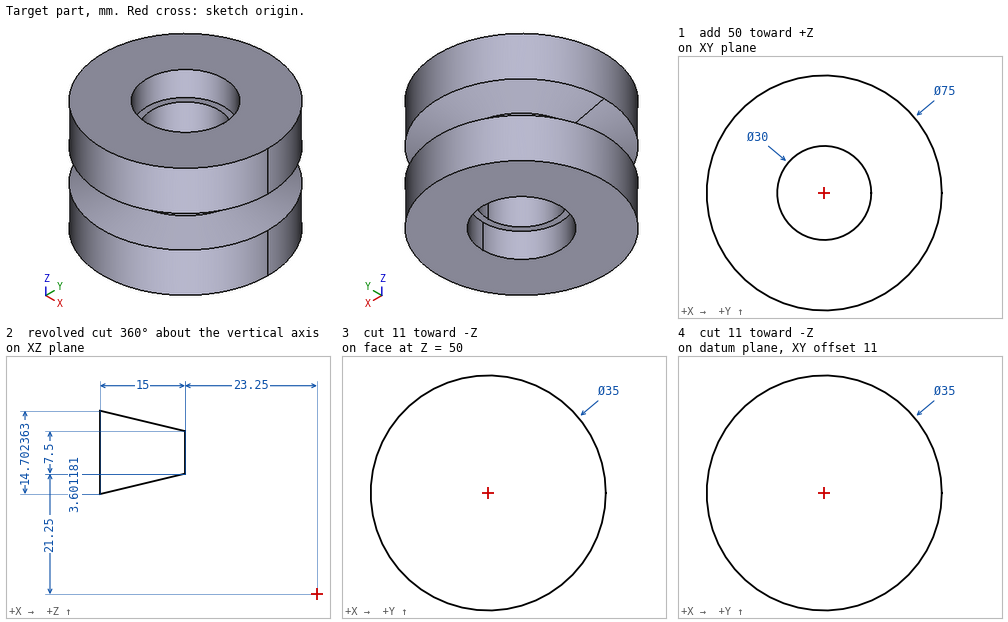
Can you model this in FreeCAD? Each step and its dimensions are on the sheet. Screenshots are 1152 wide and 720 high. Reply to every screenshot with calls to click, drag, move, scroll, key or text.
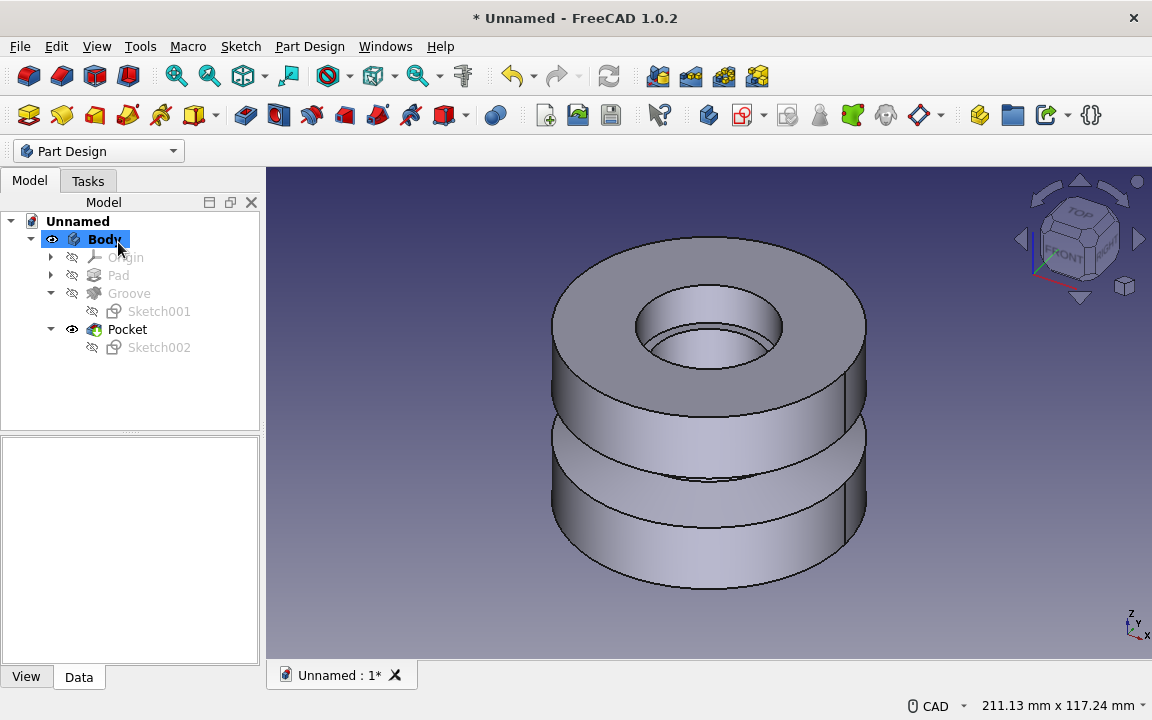
click(51, 257)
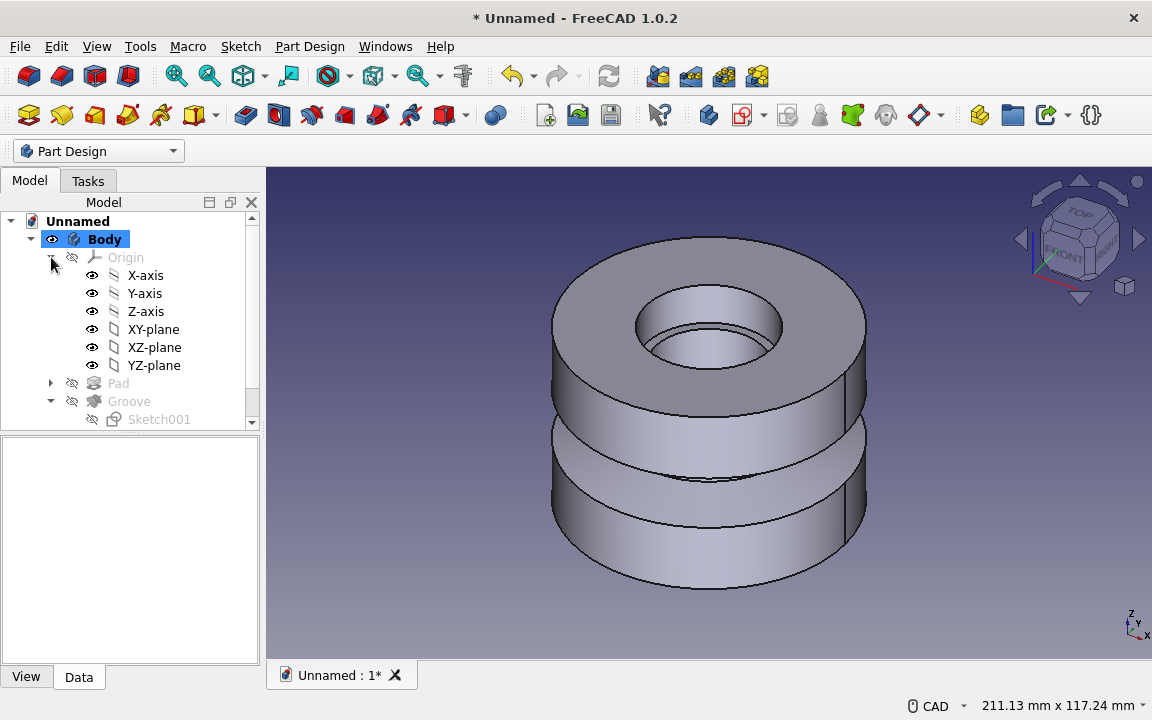
click(137, 329)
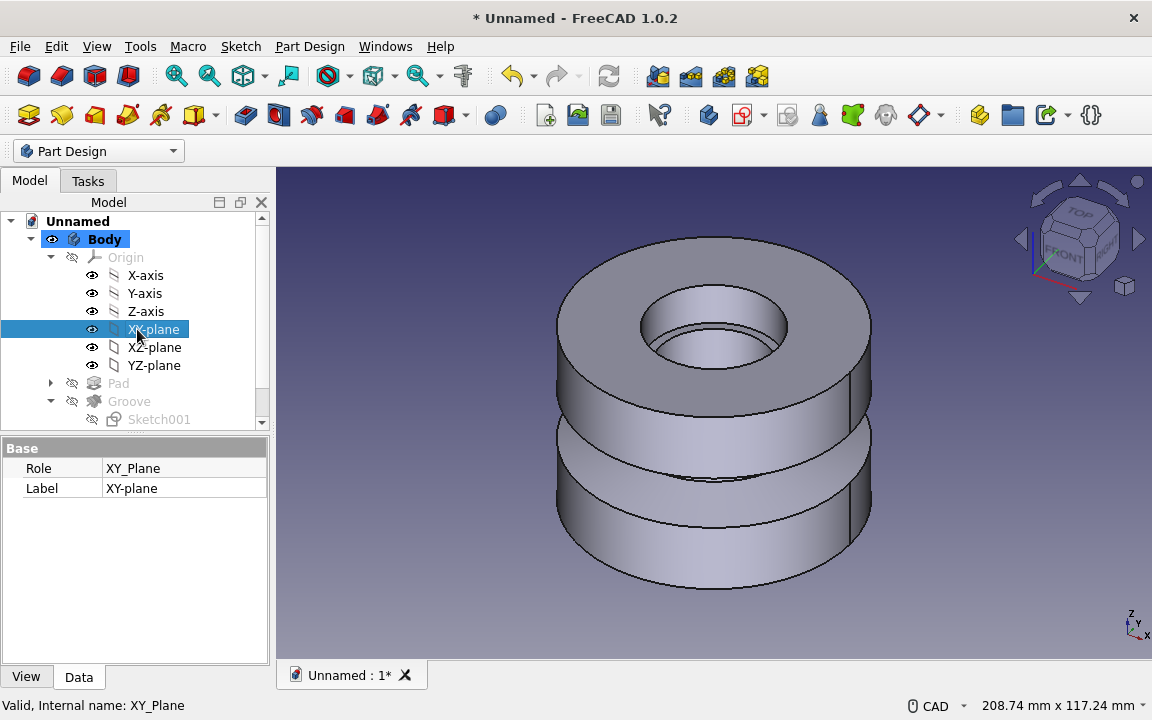
click(918, 116)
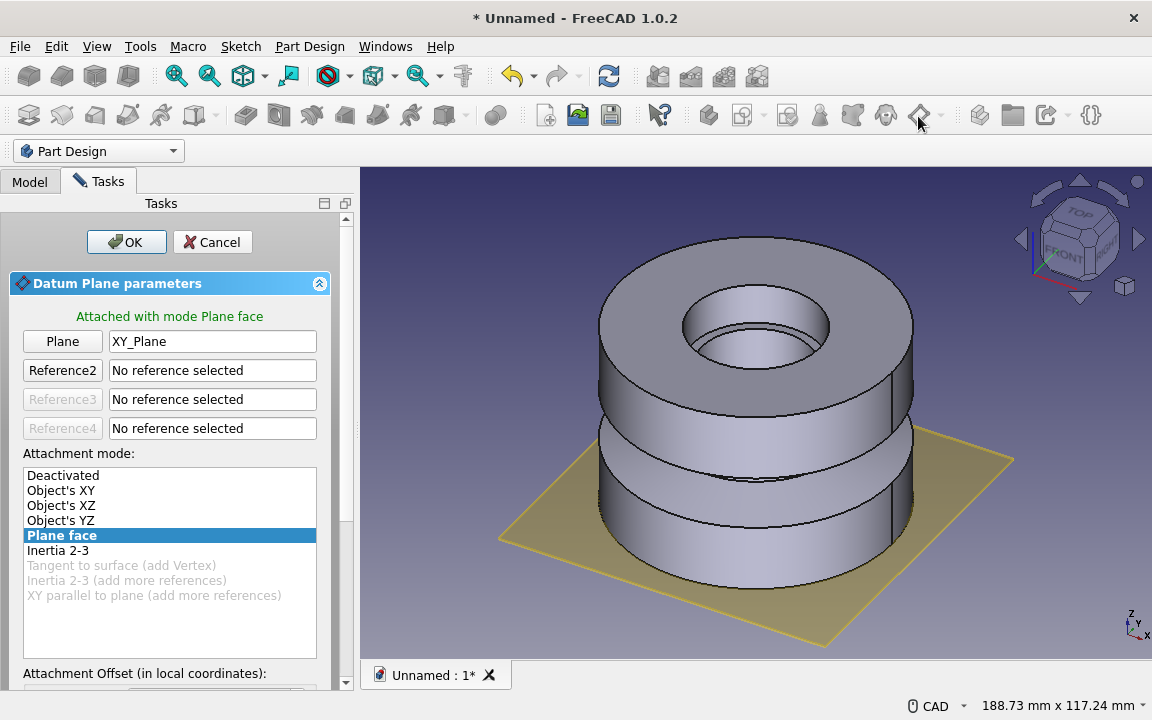
scroll(346, 452, down, 3)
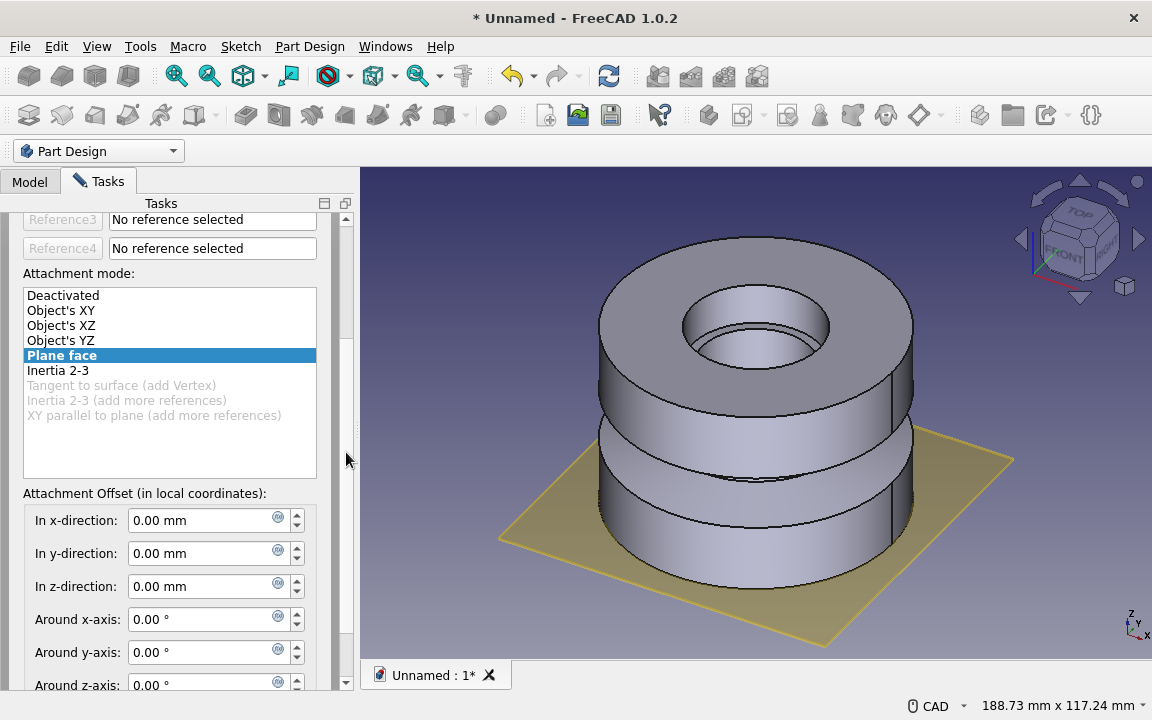
triple_click(210, 586)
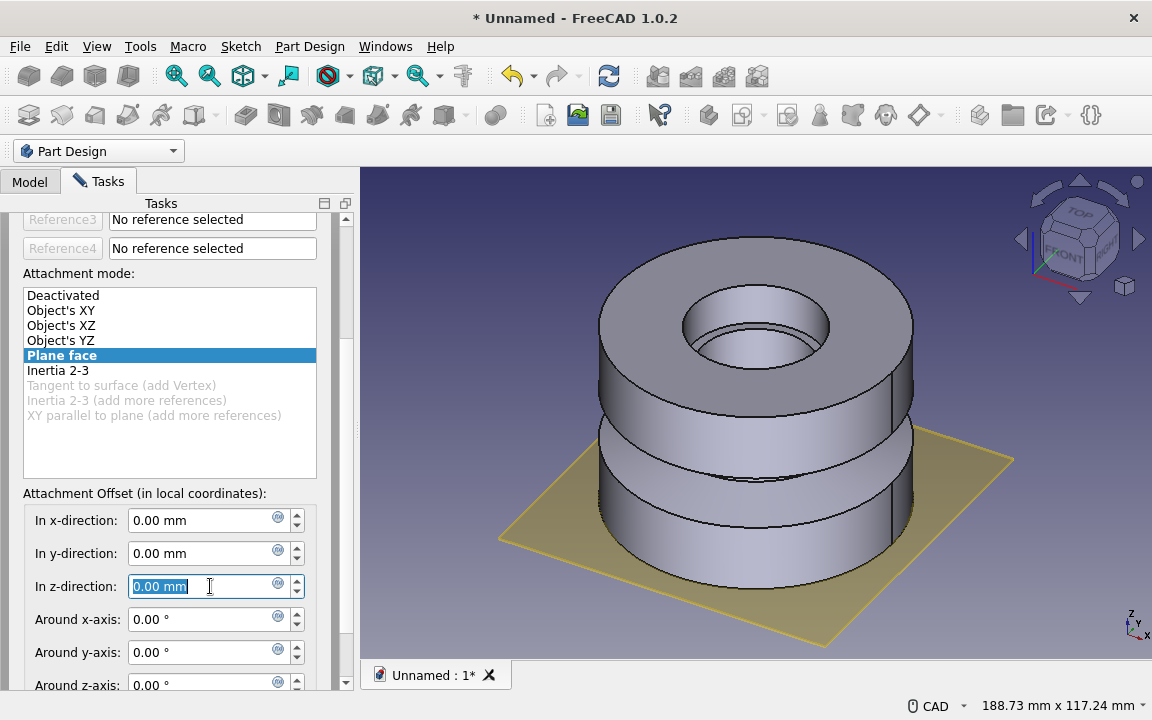
text(11)
key(Tab)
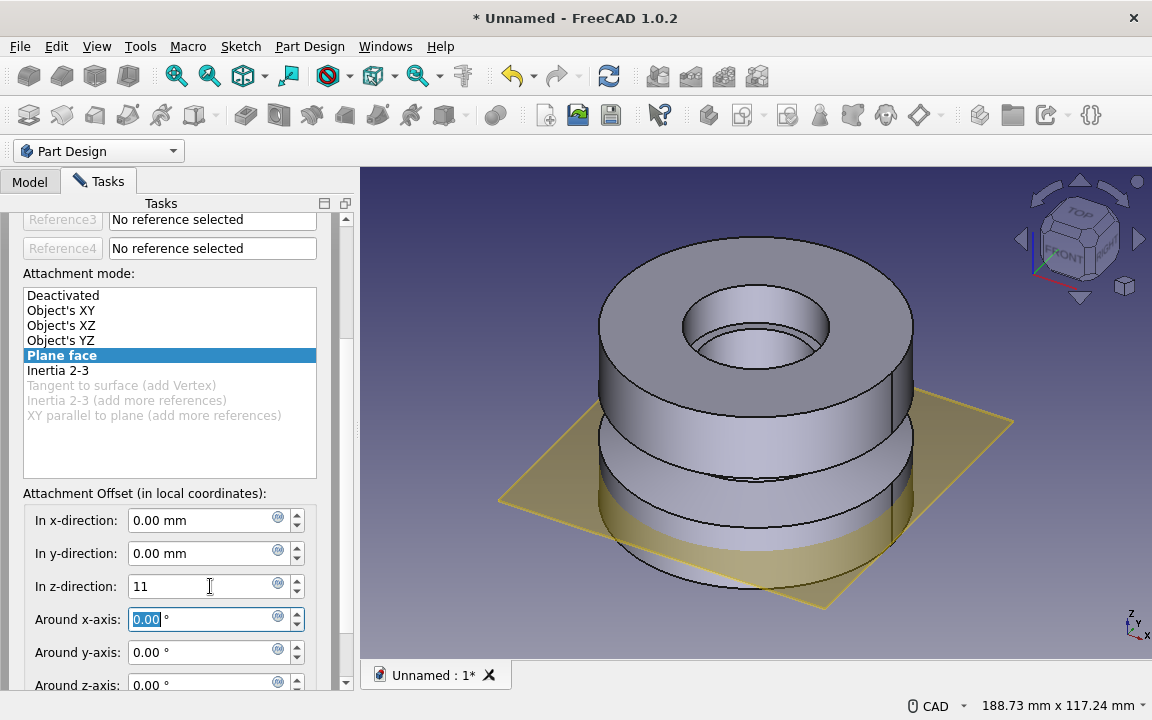
scroll(346, 452, up, 4)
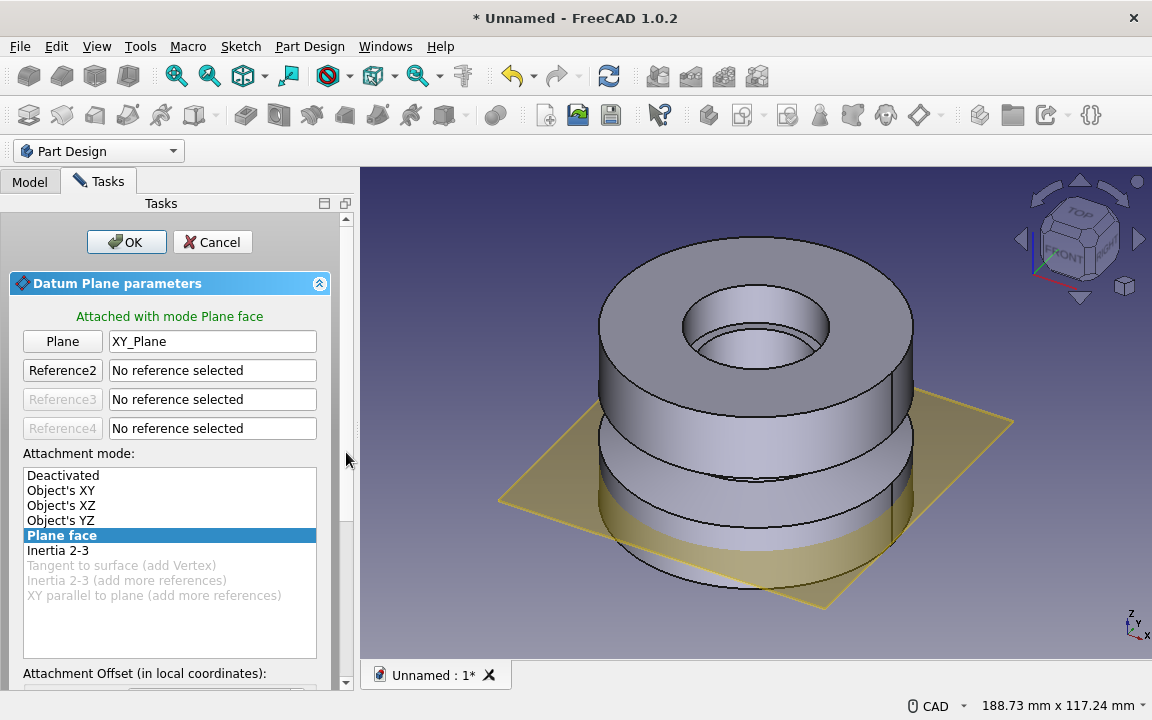
click(127, 242)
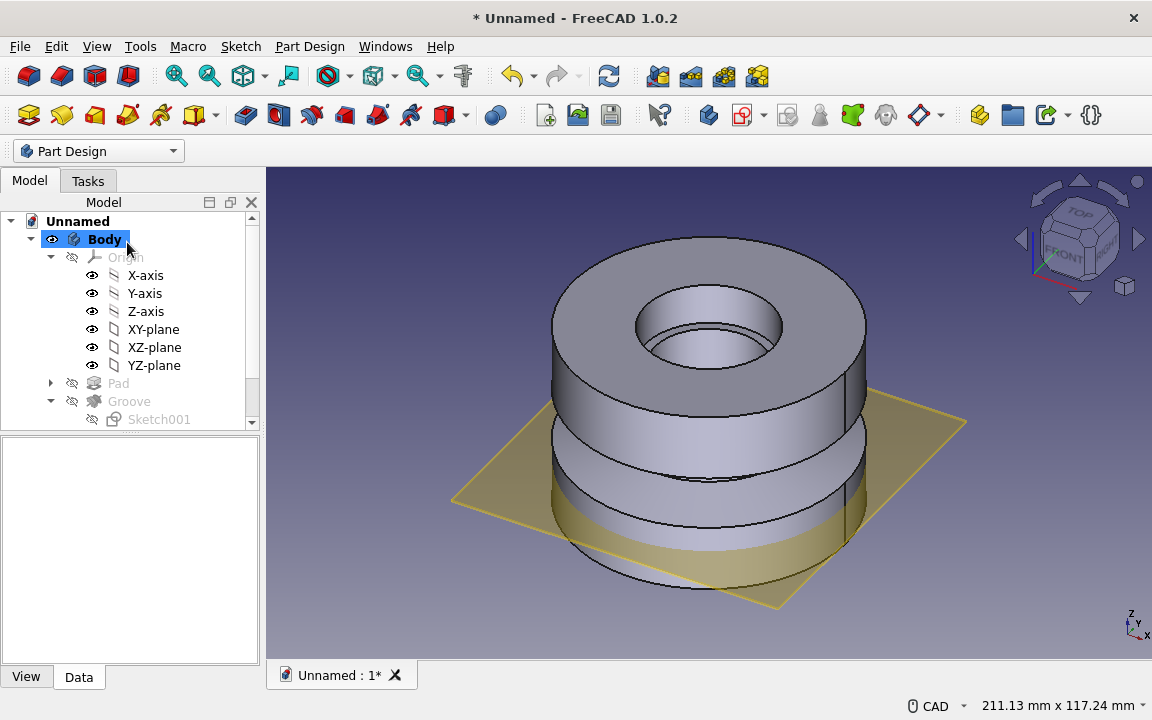
scroll(101, 325, down, 3)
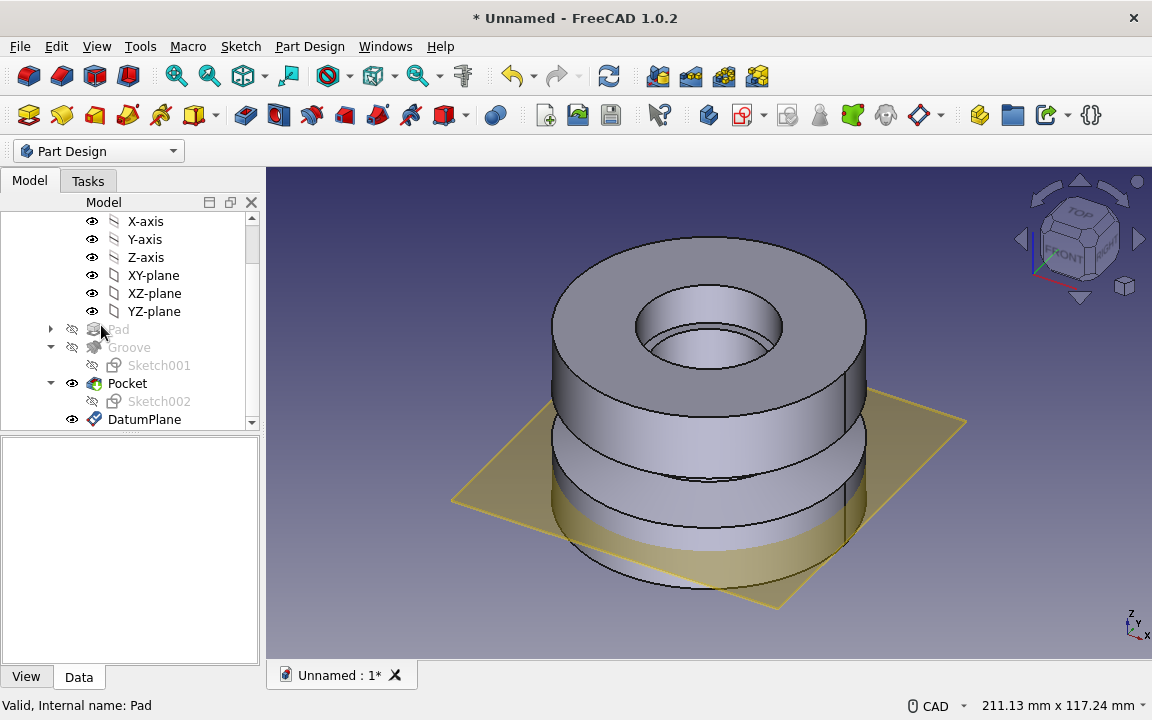
click(117, 419)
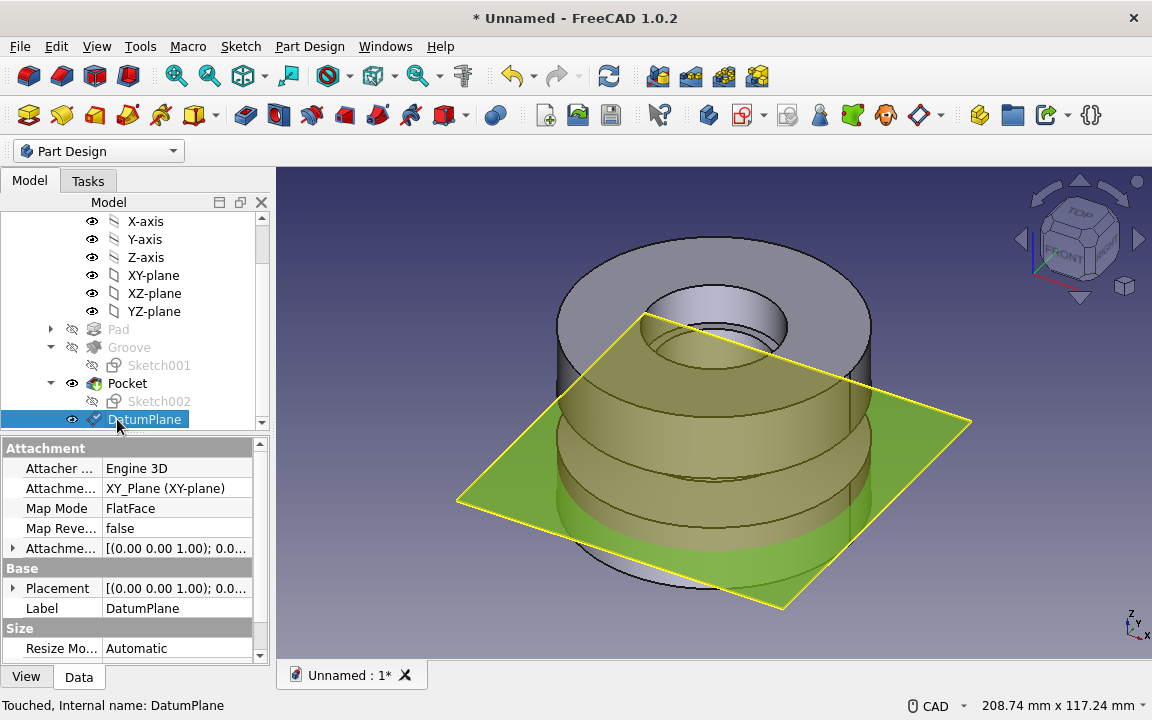
click(742, 116)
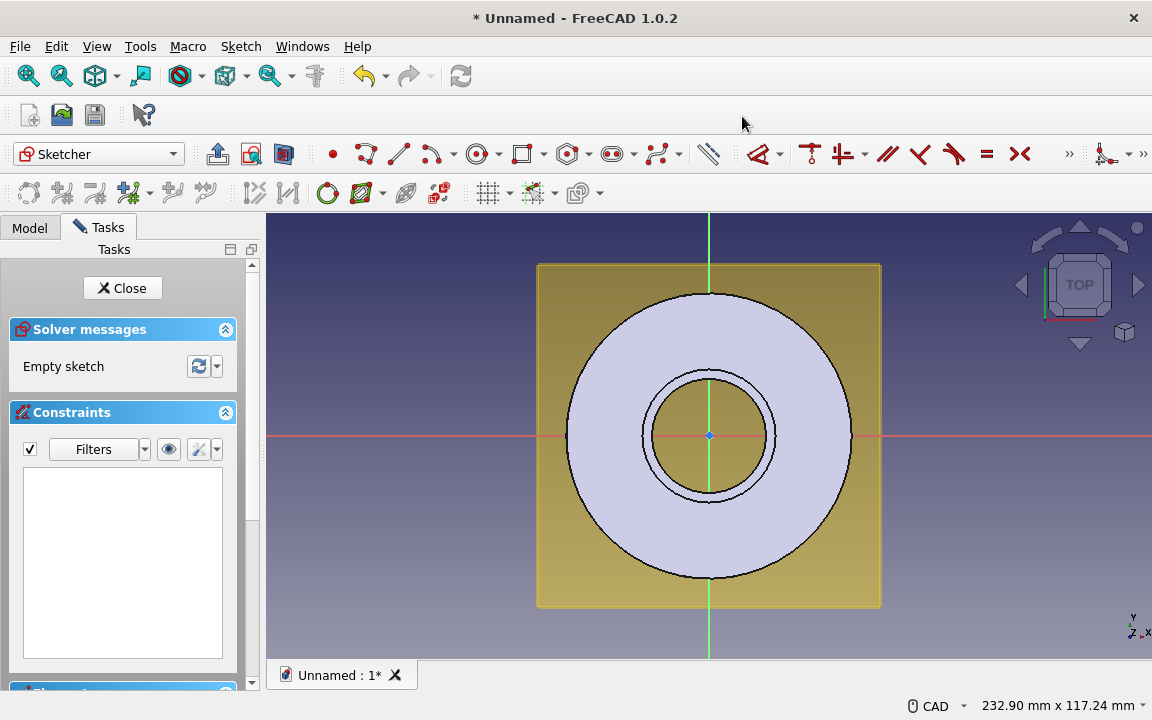
key(q)
key(s)